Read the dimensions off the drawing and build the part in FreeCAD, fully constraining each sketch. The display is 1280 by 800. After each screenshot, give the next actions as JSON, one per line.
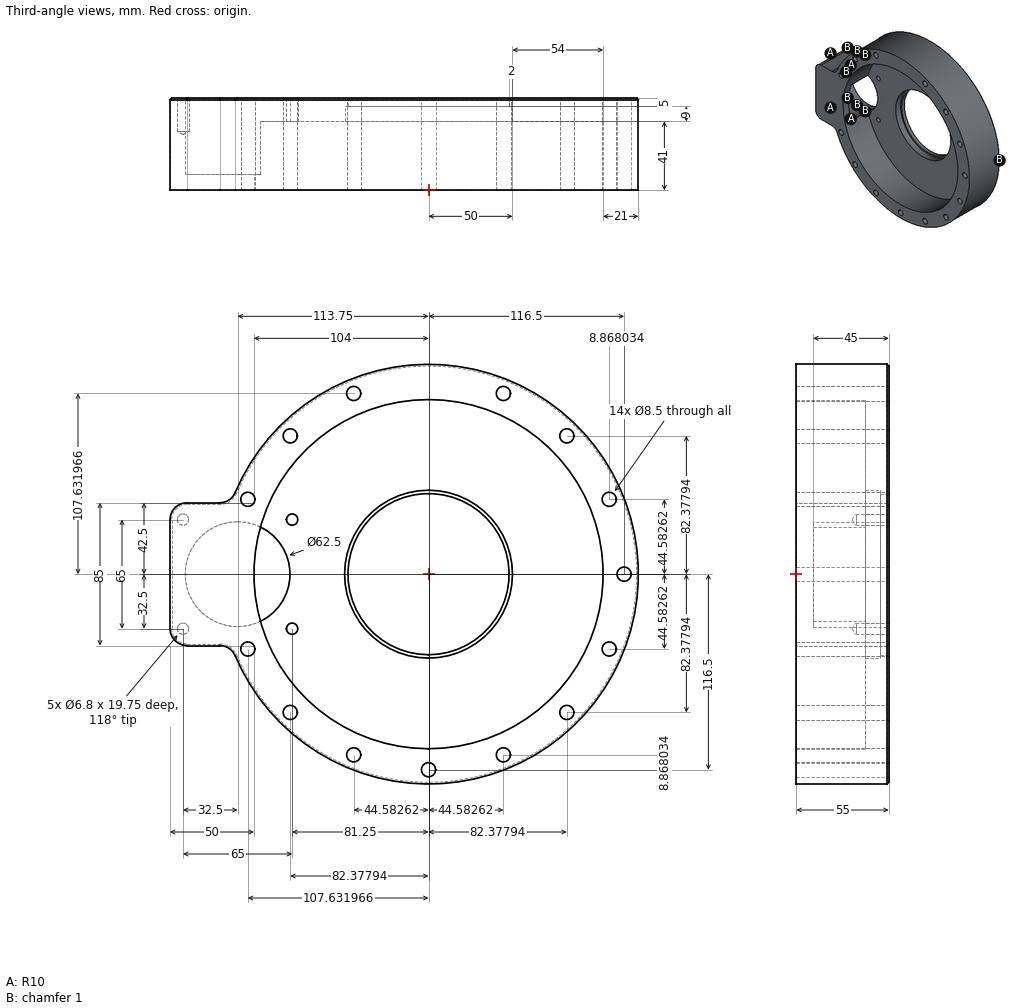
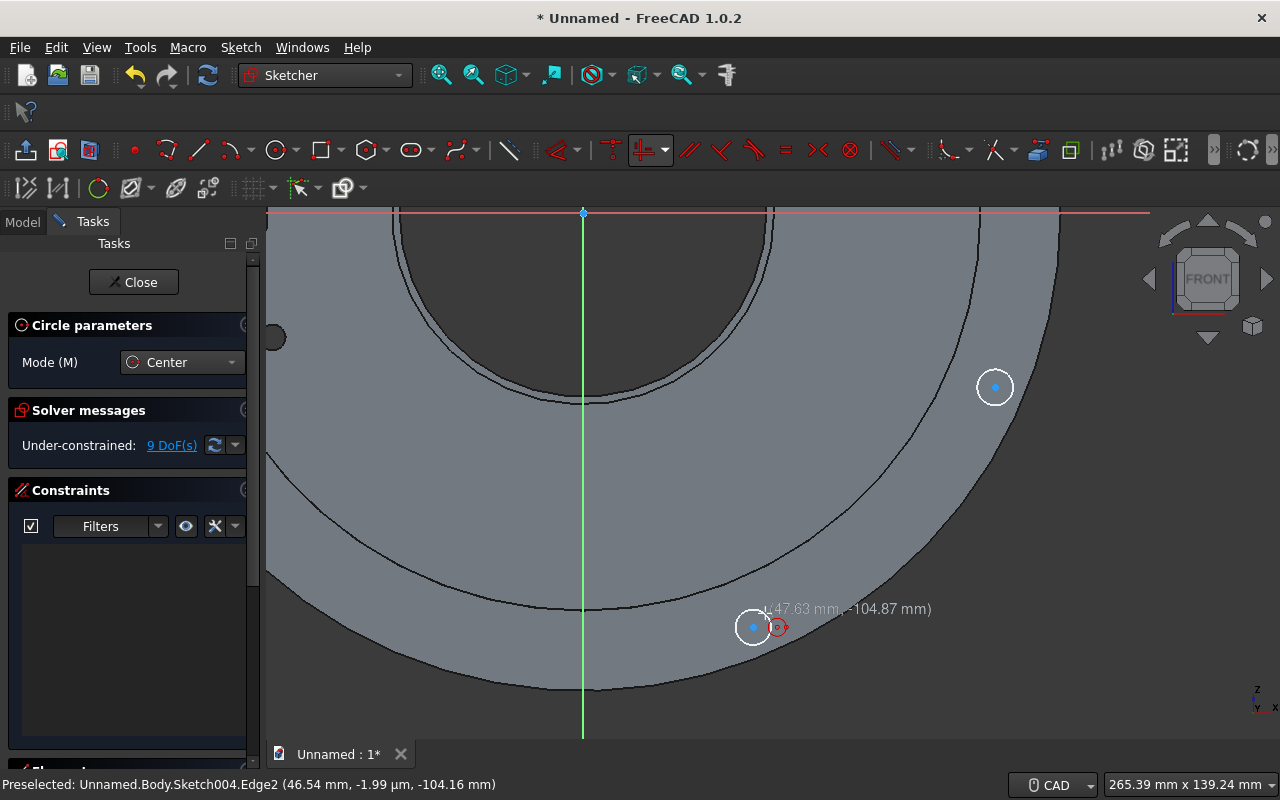
{"action": "scroll", "coordinate": [413, 625], "scroll_direction": "up", "scroll_amount": 2}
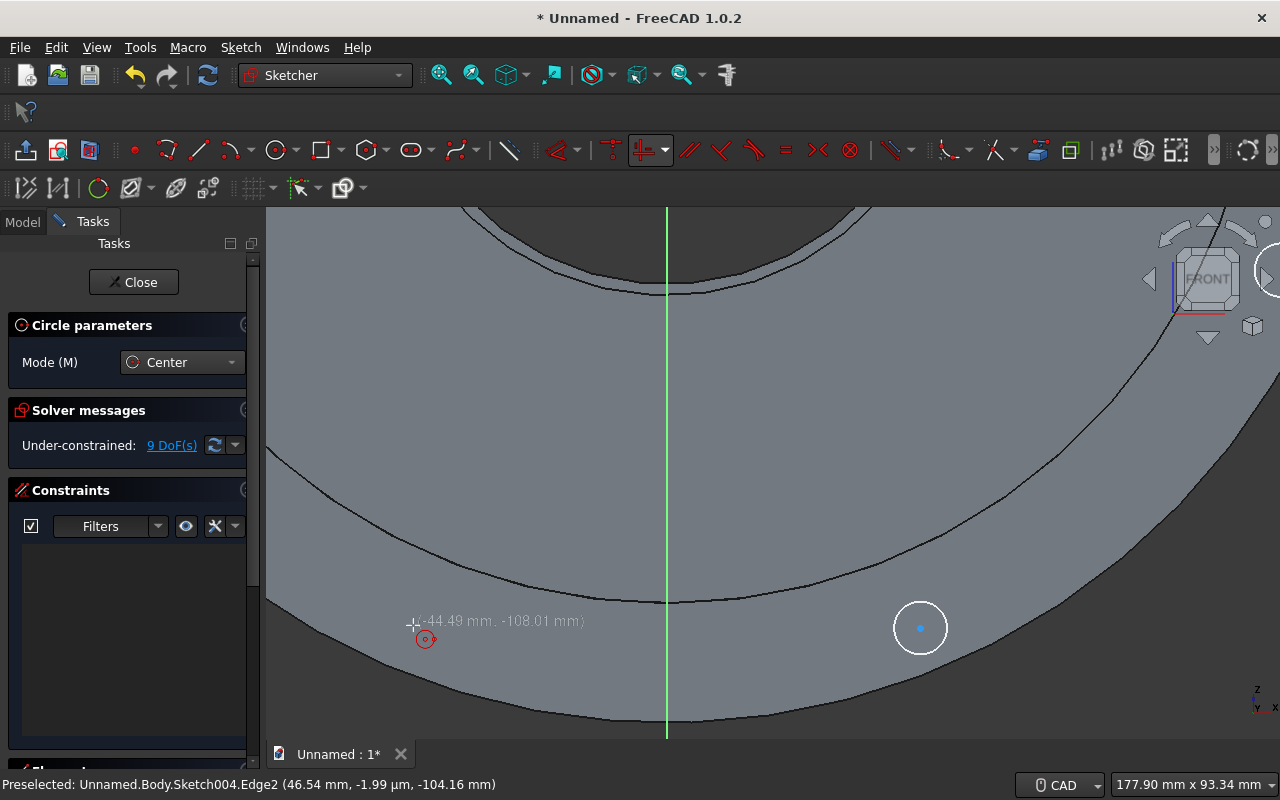
{"action": "scroll", "coordinate": [709, 616], "scroll_direction": "down", "scroll_amount": 7}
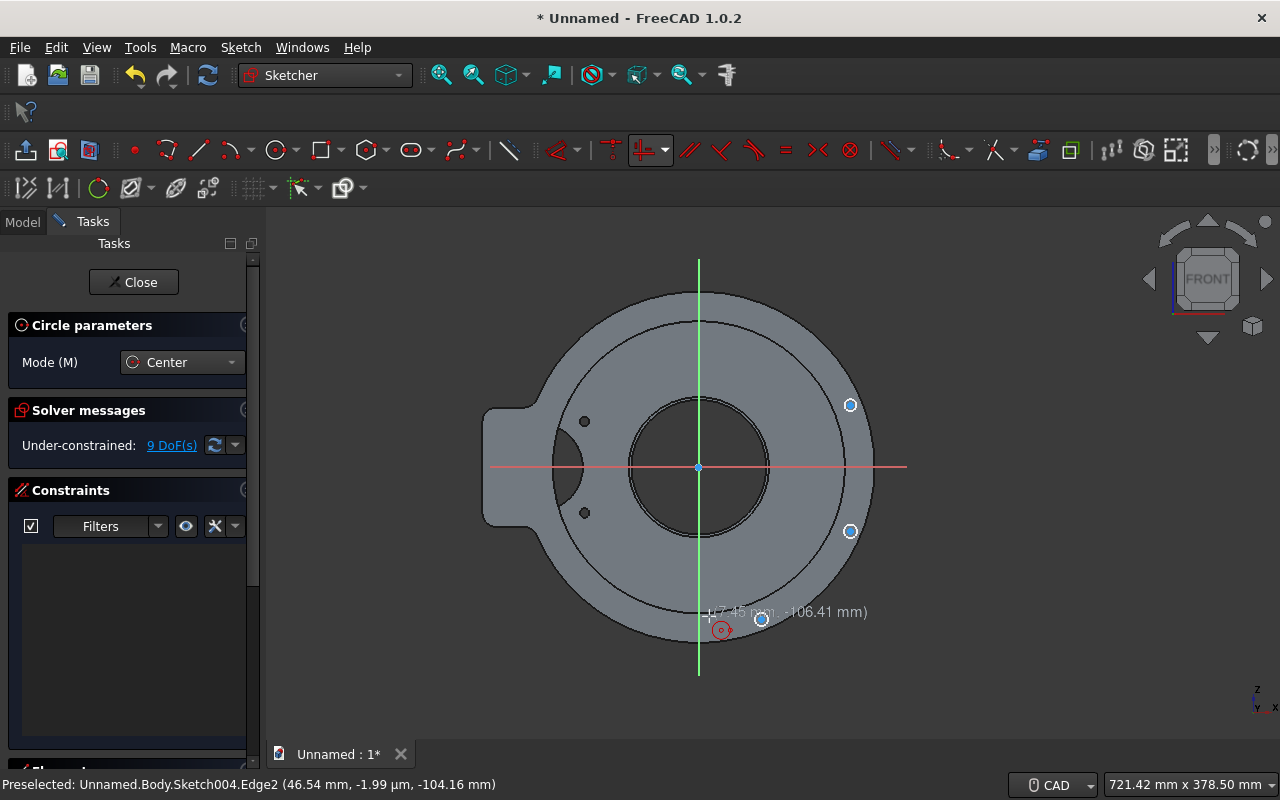
{"action": "left_click", "coordinate": [636, 619]}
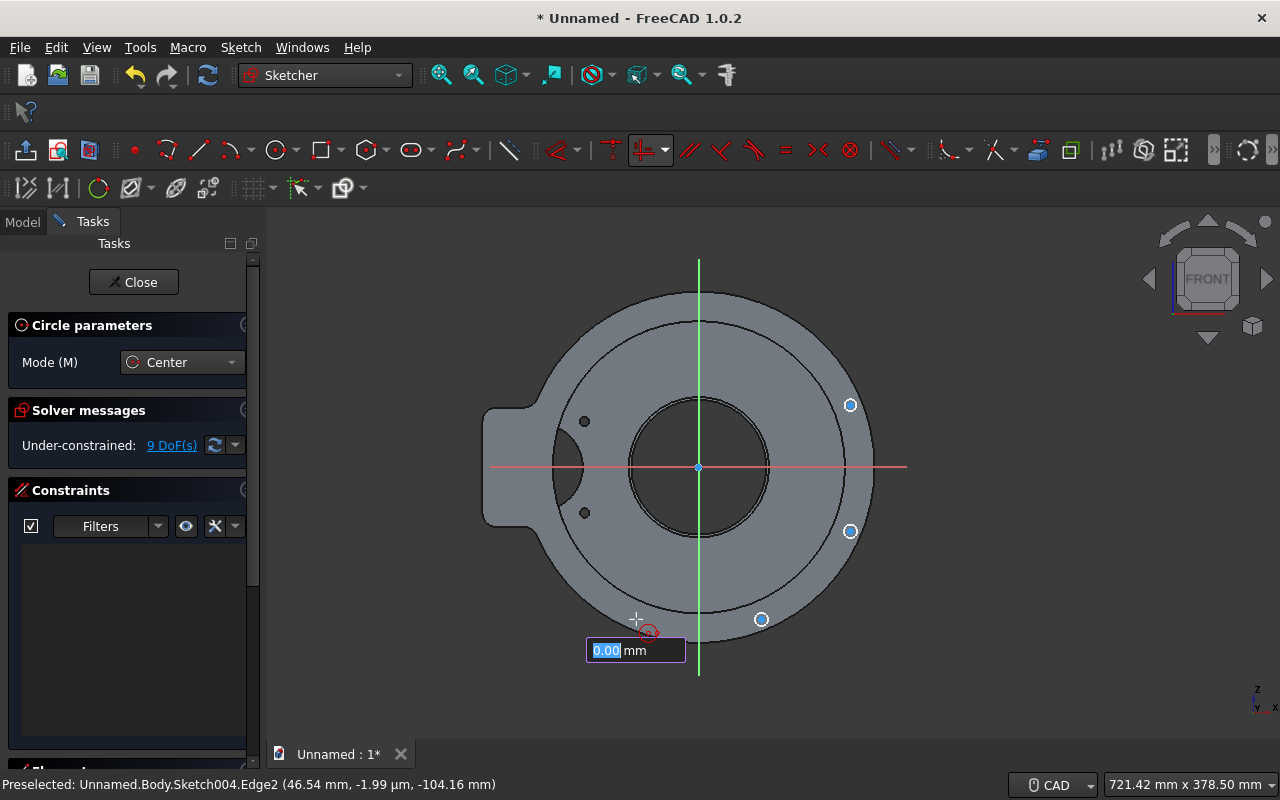
{"action": "scroll", "coordinate": [640, 614], "scroll_direction": "up", "scroll_amount": 5}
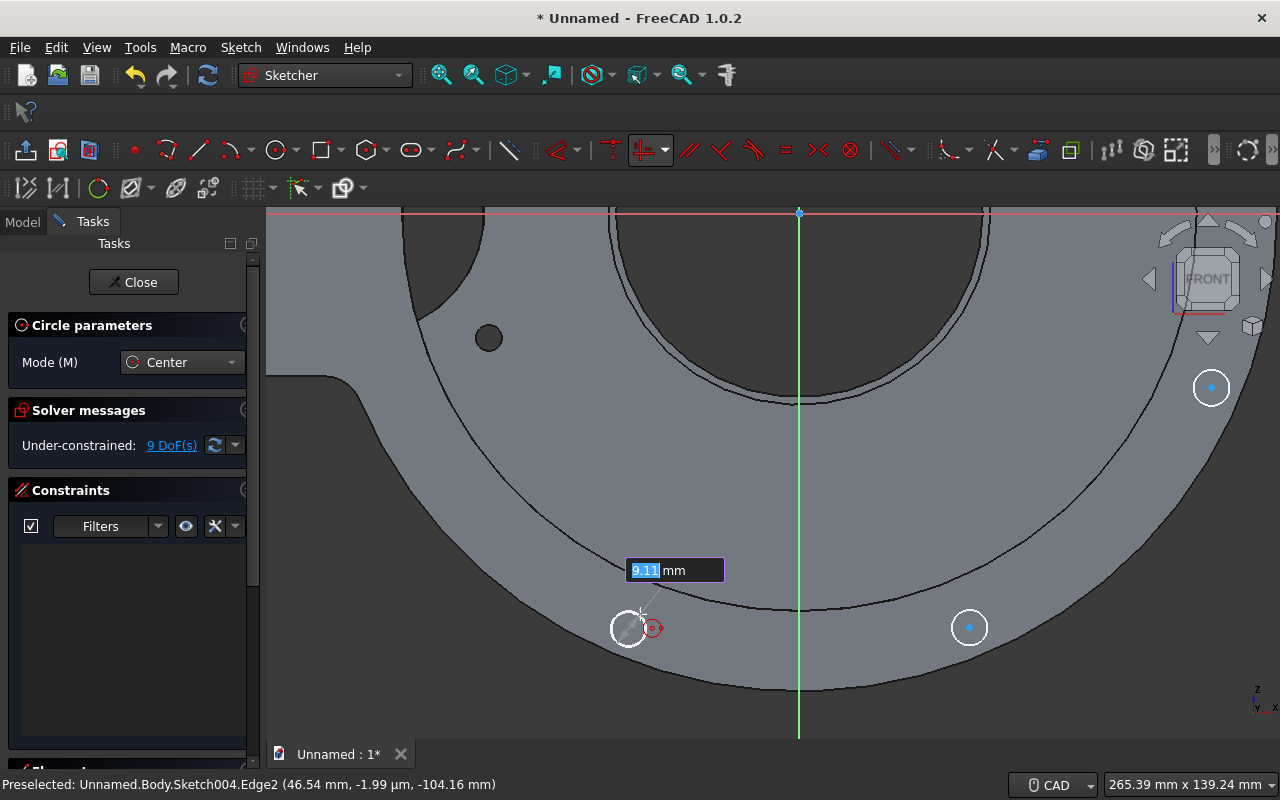
{"action": "left_click", "coordinate": [641, 614]}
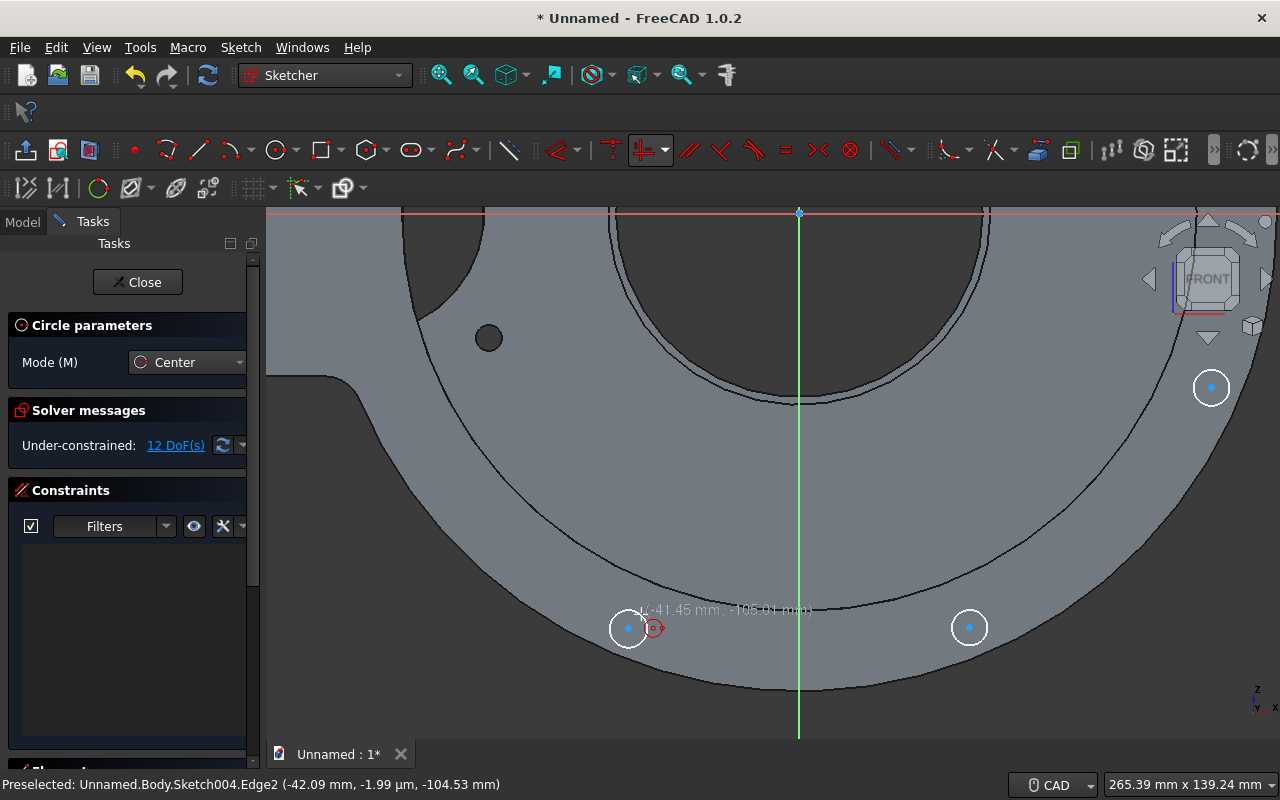
{"action": "scroll", "coordinate": [388, 384], "scroll_direction": "up", "scroll_amount": 2}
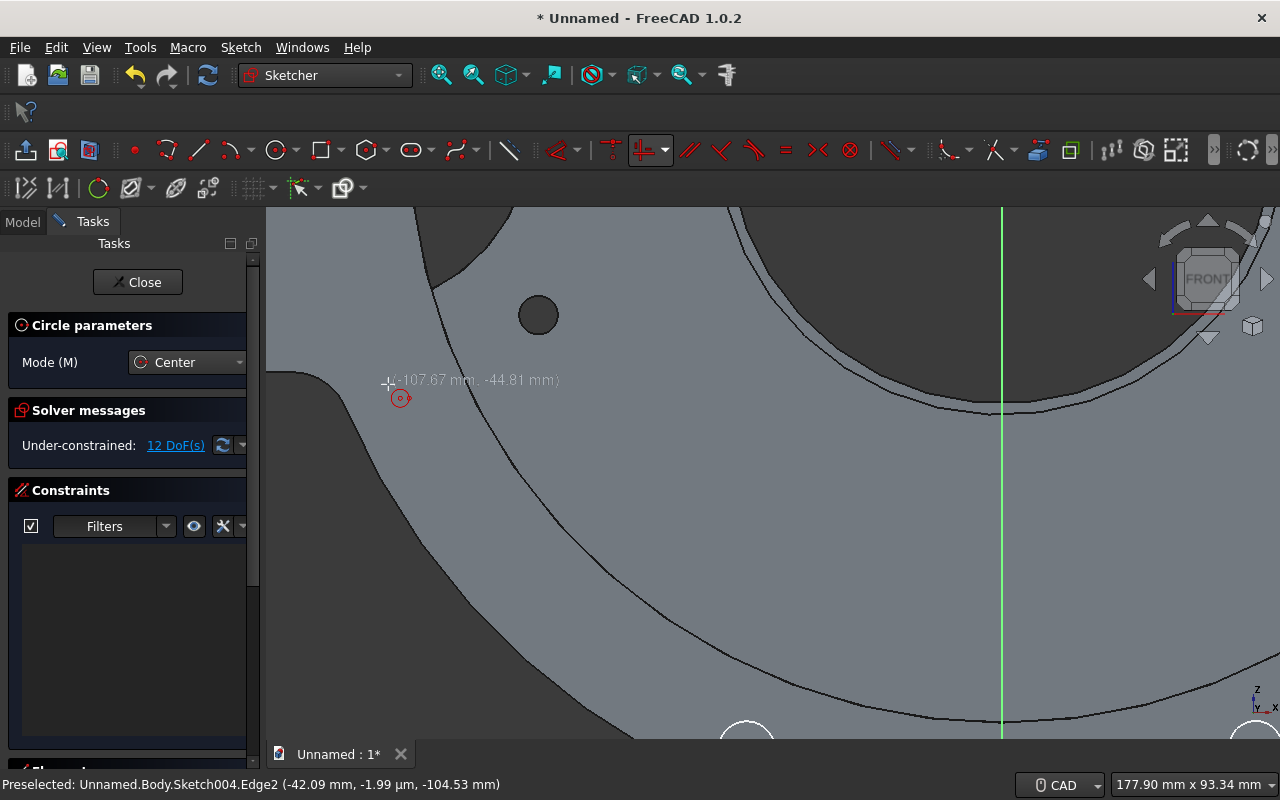
{"action": "scroll", "coordinate": [599, 577], "scroll_direction": "down", "scroll_amount": 7}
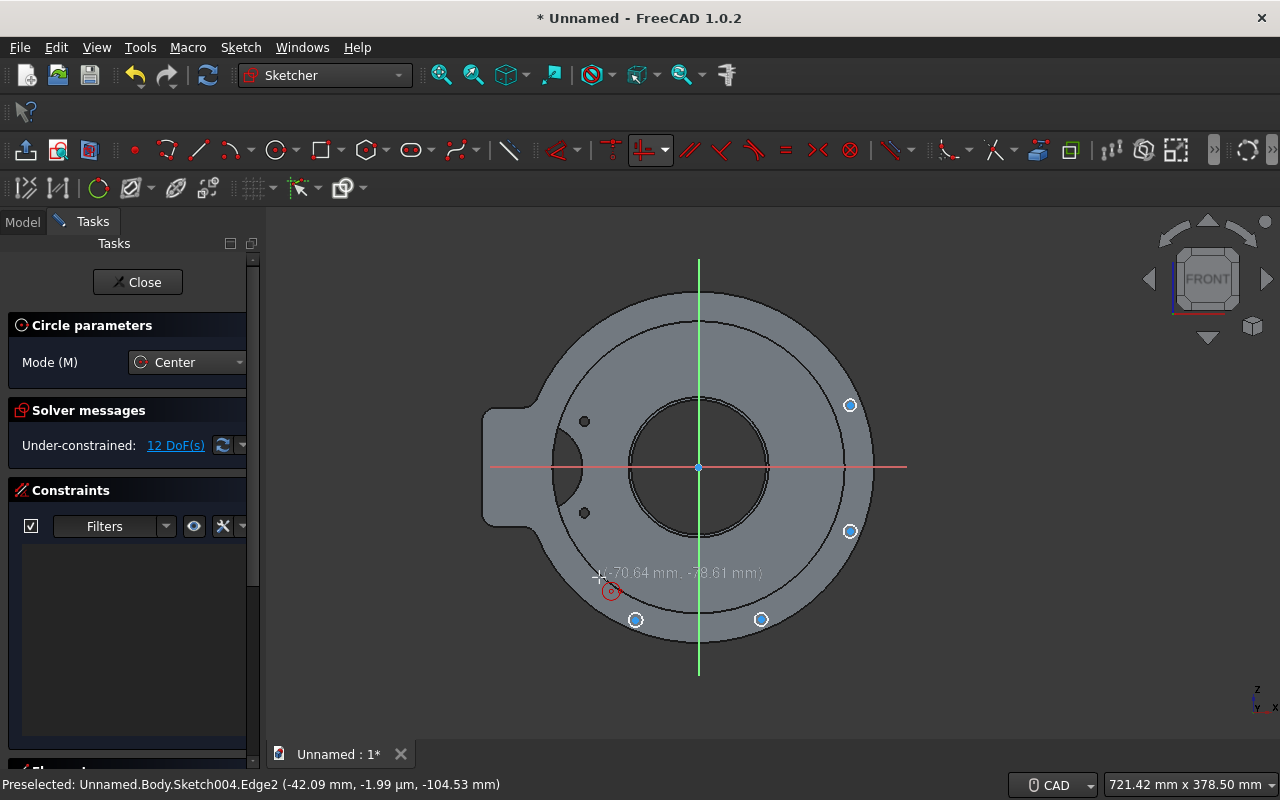
{"action": "left_click", "coordinate": [547, 530]}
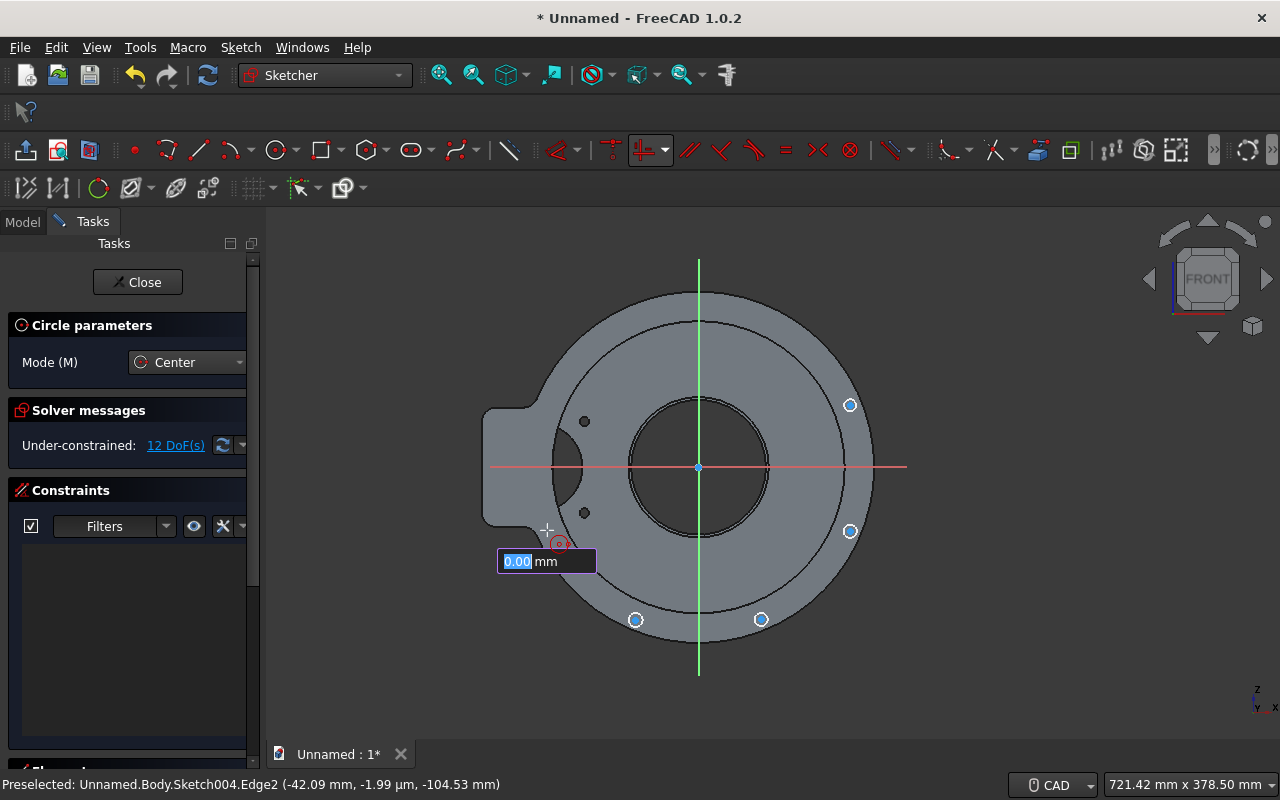
{"action": "scroll", "coordinate": [551, 526], "scroll_direction": "up", "scroll_amount": 5}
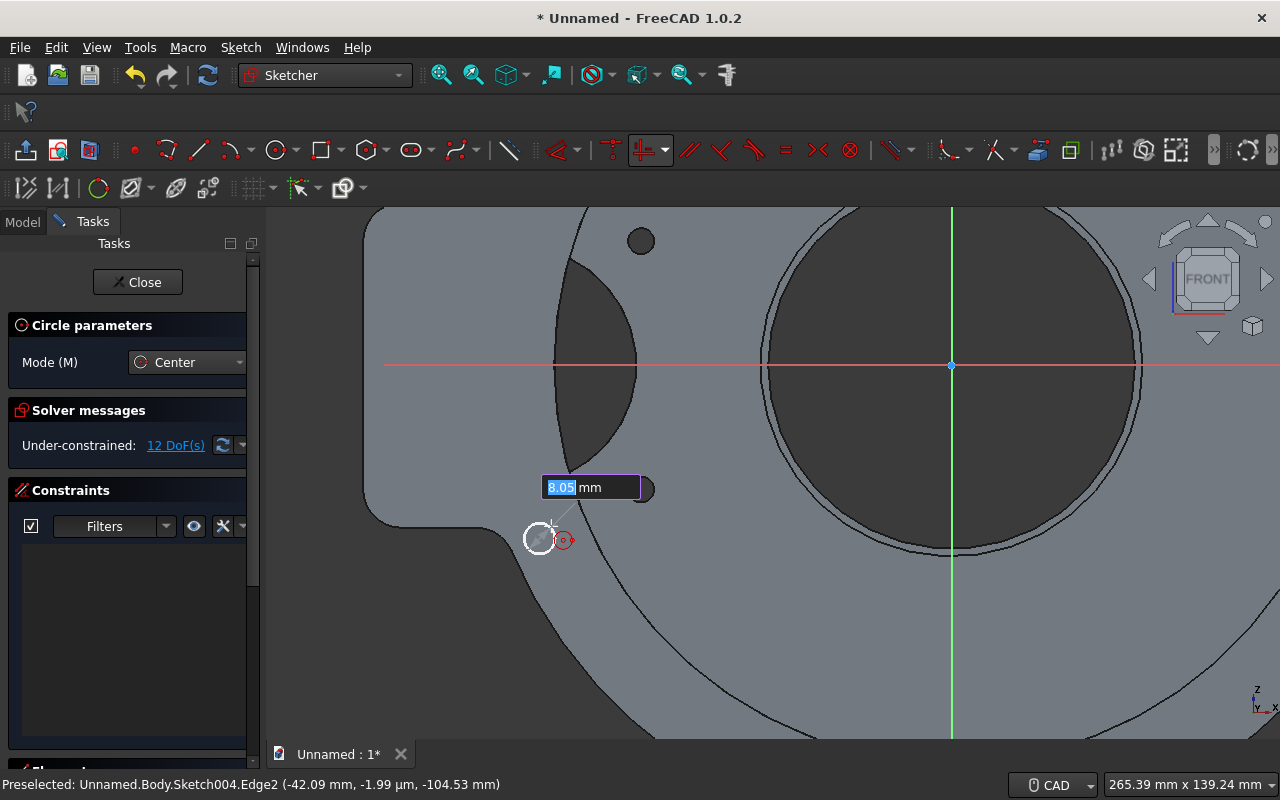
{"action": "left_click", "coordinate": [552, 524]}